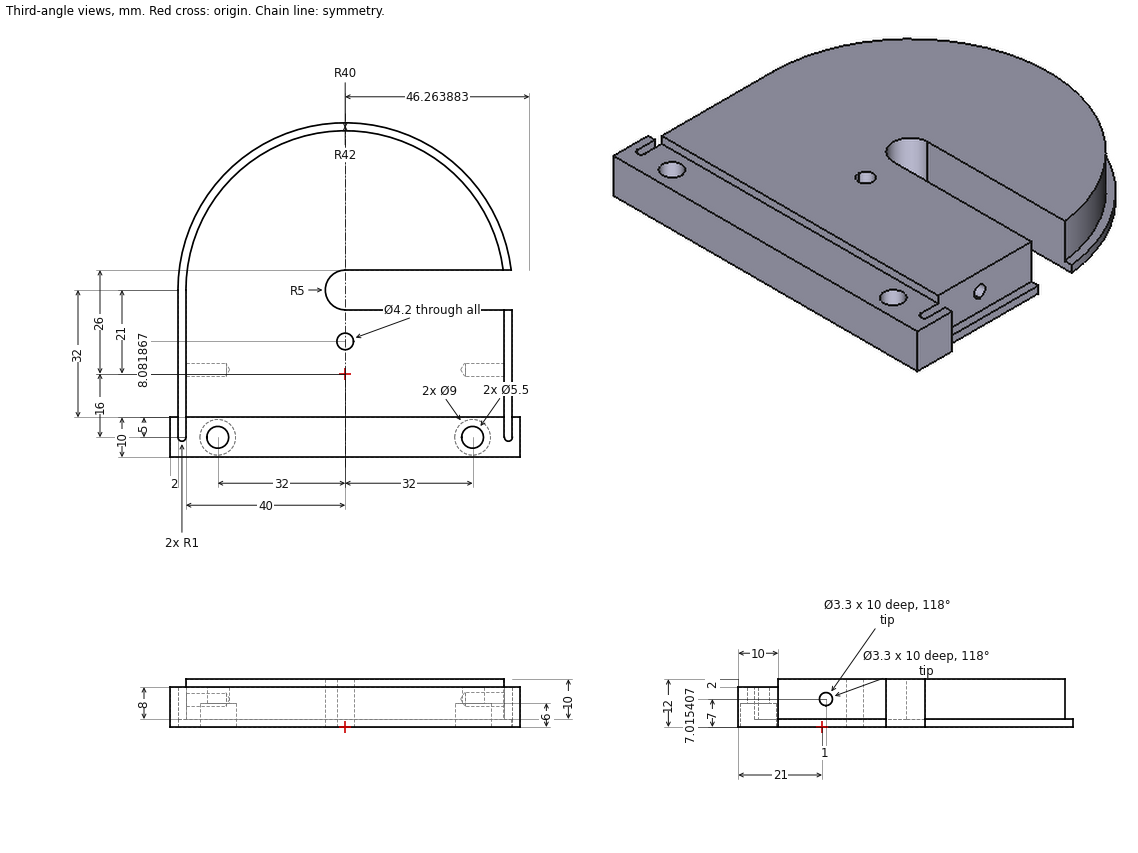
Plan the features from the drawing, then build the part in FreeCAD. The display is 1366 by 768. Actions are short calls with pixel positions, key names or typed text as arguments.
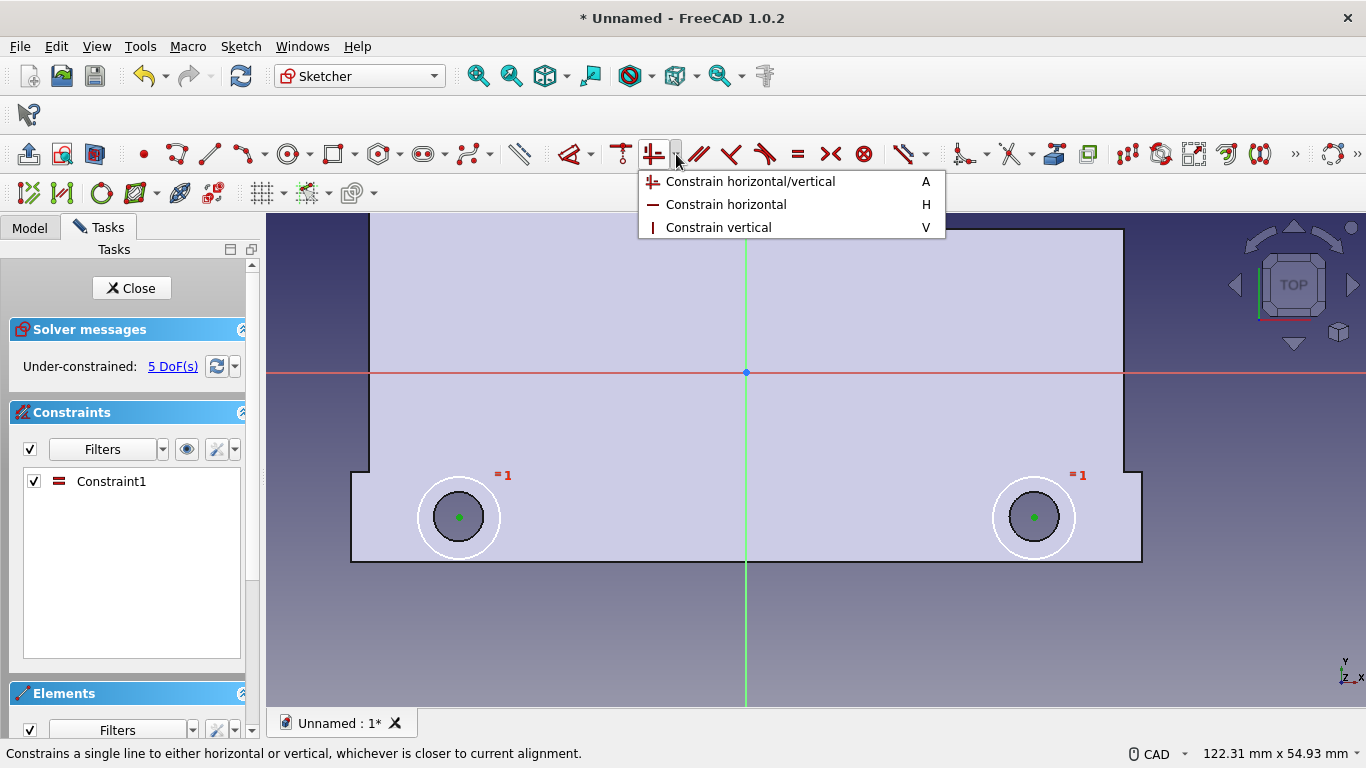
click(792, 204)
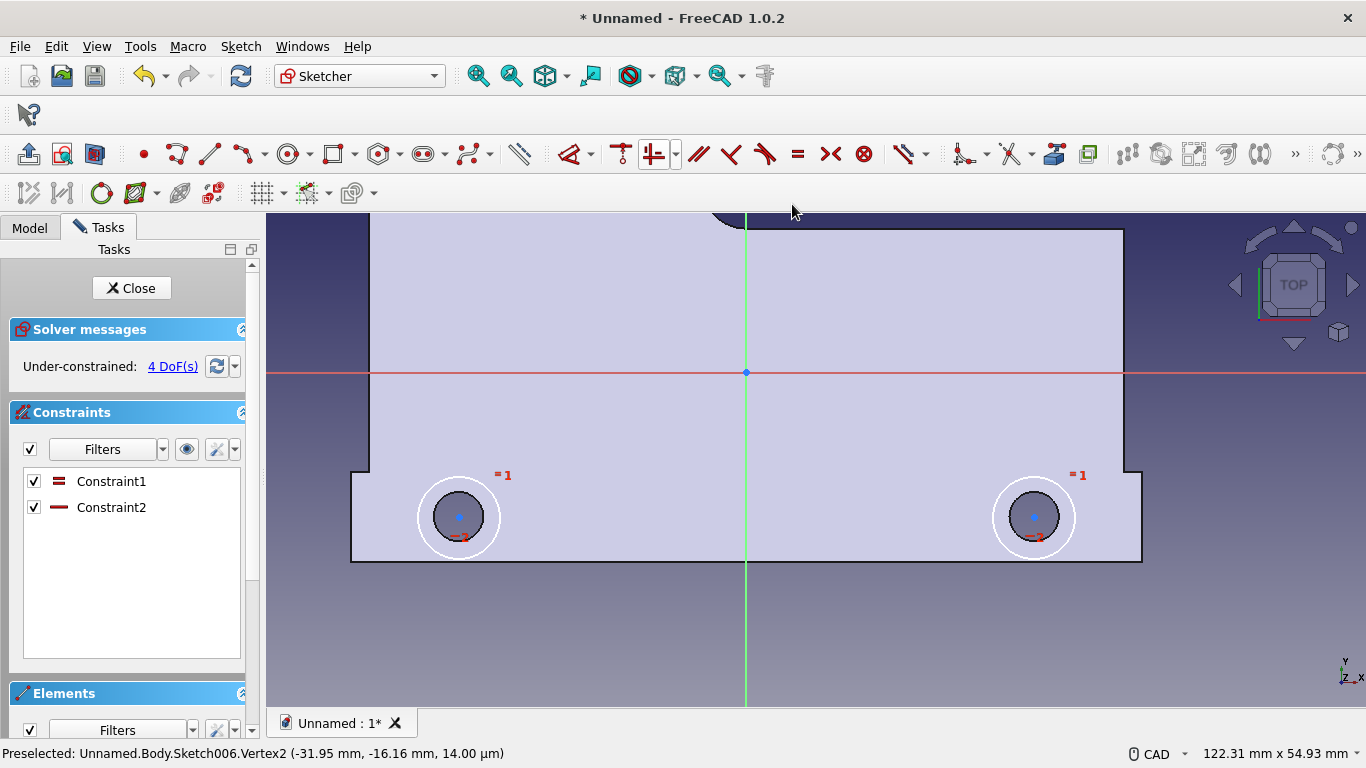
key(d)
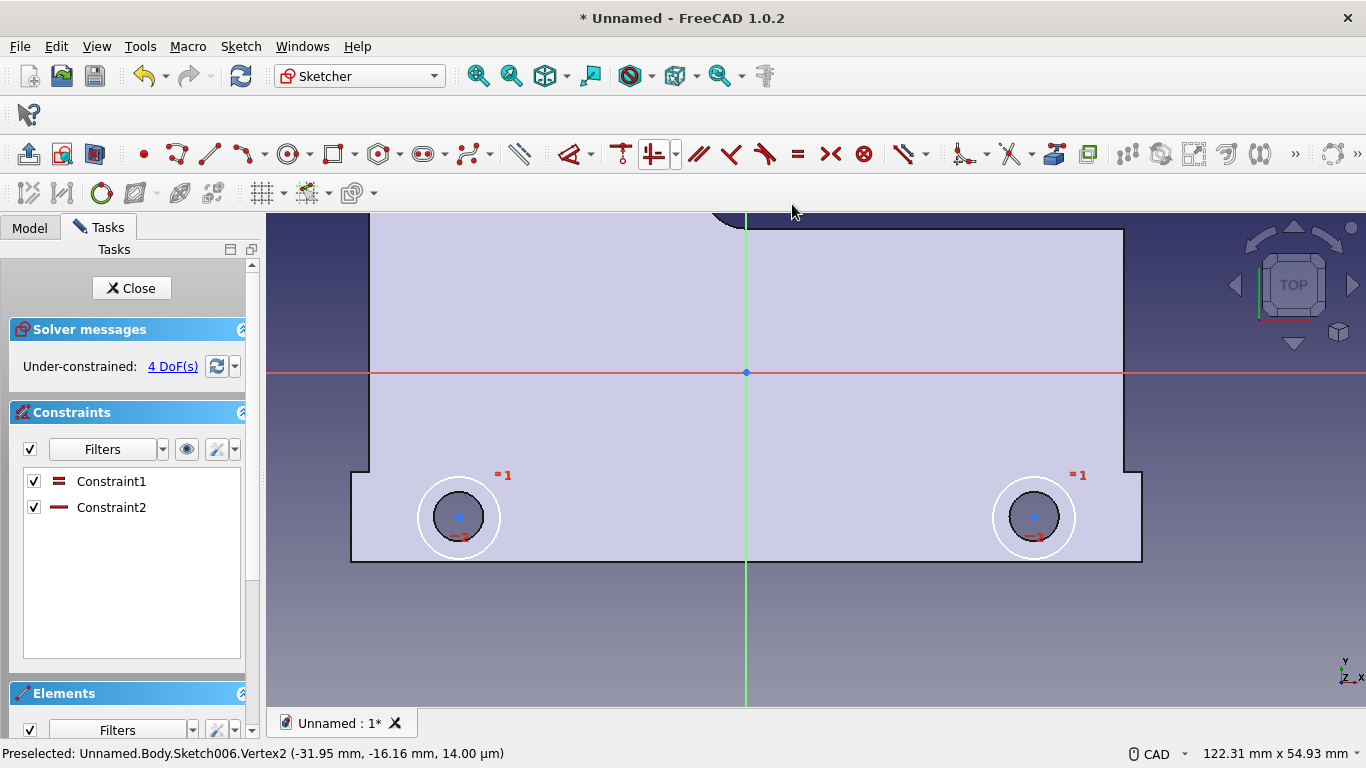
click(1063, 489)
click(1086, 466)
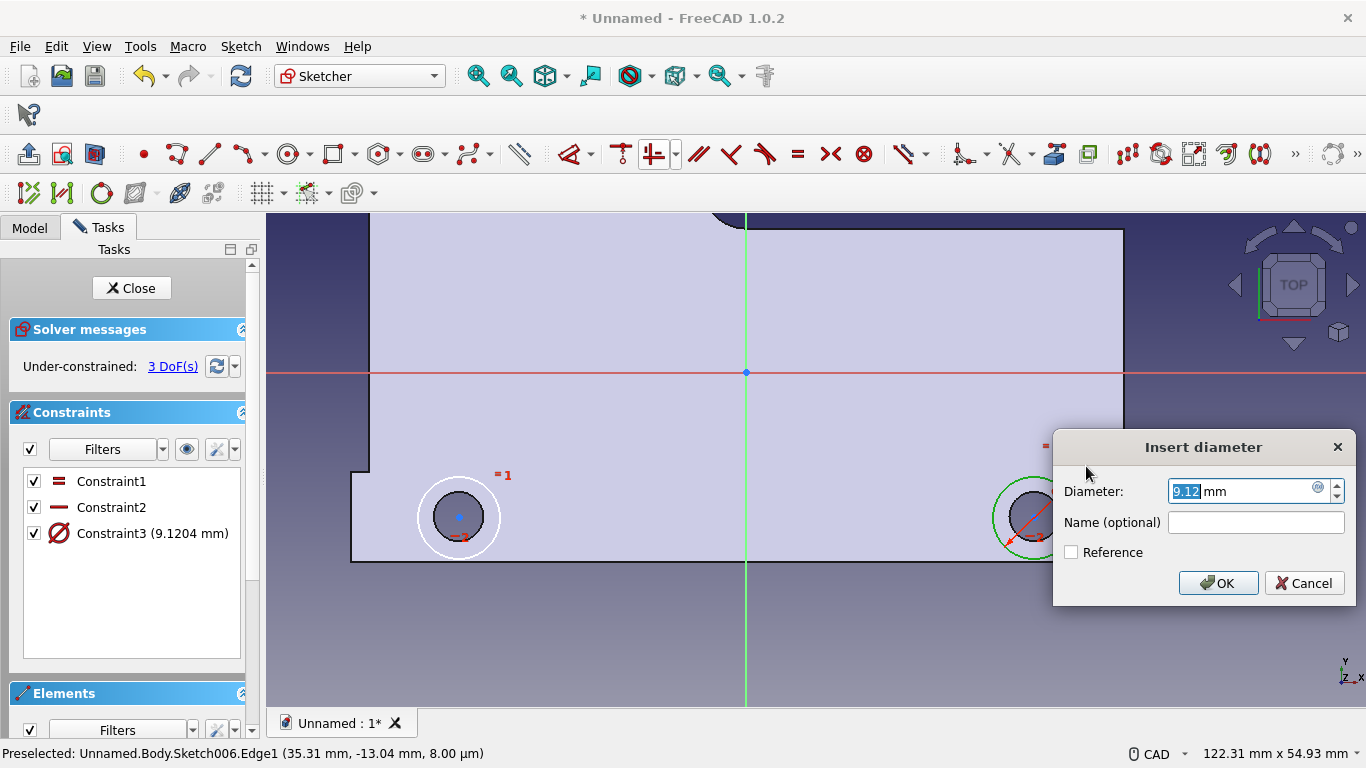
text(9)
key(Return)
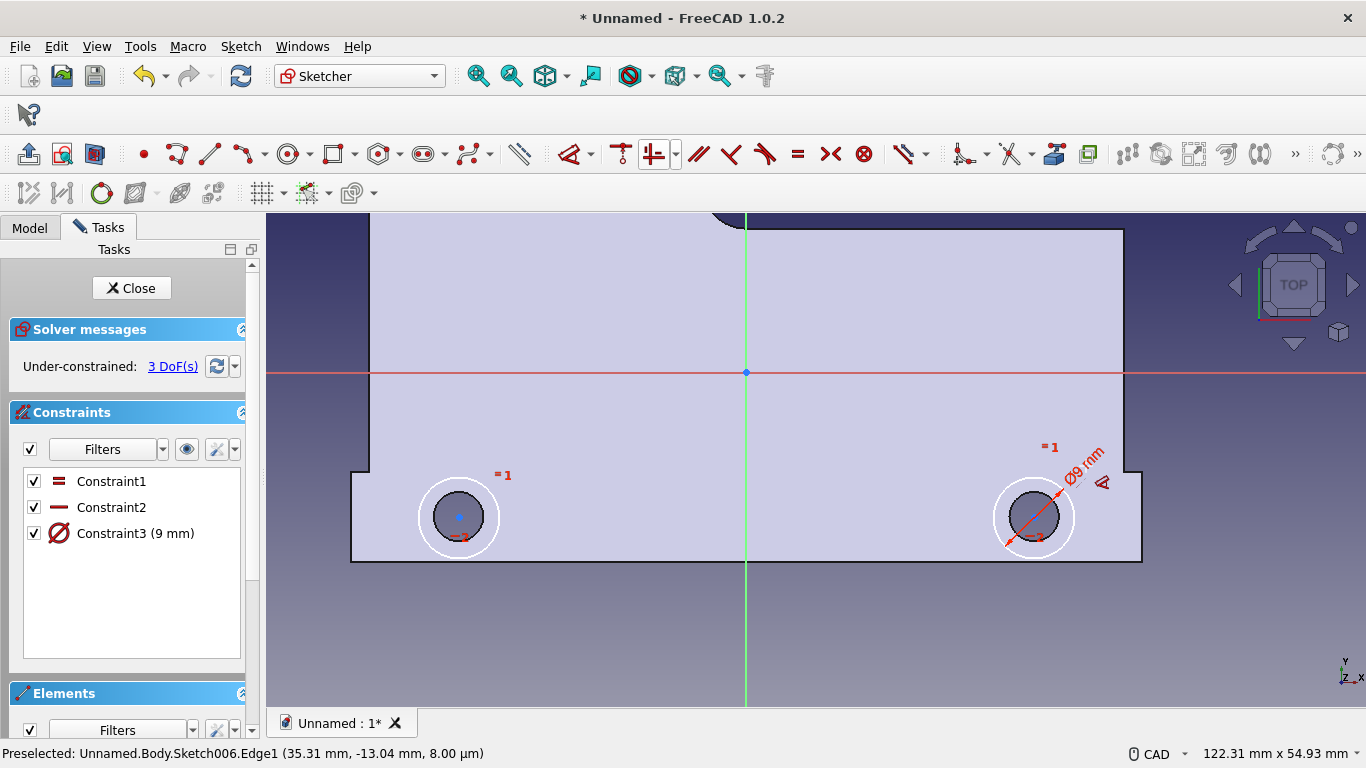
click(1034, 518)
click(890, 339)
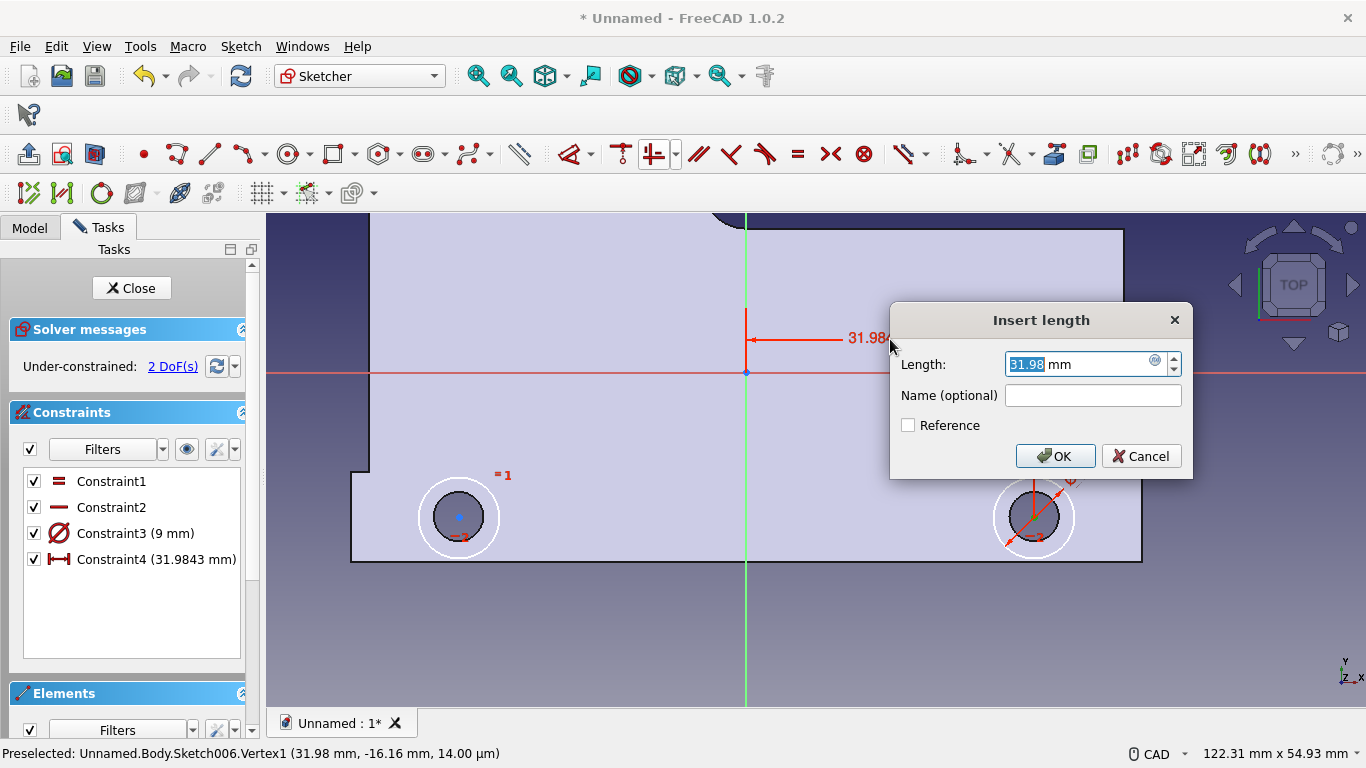
text(32)
key(Return)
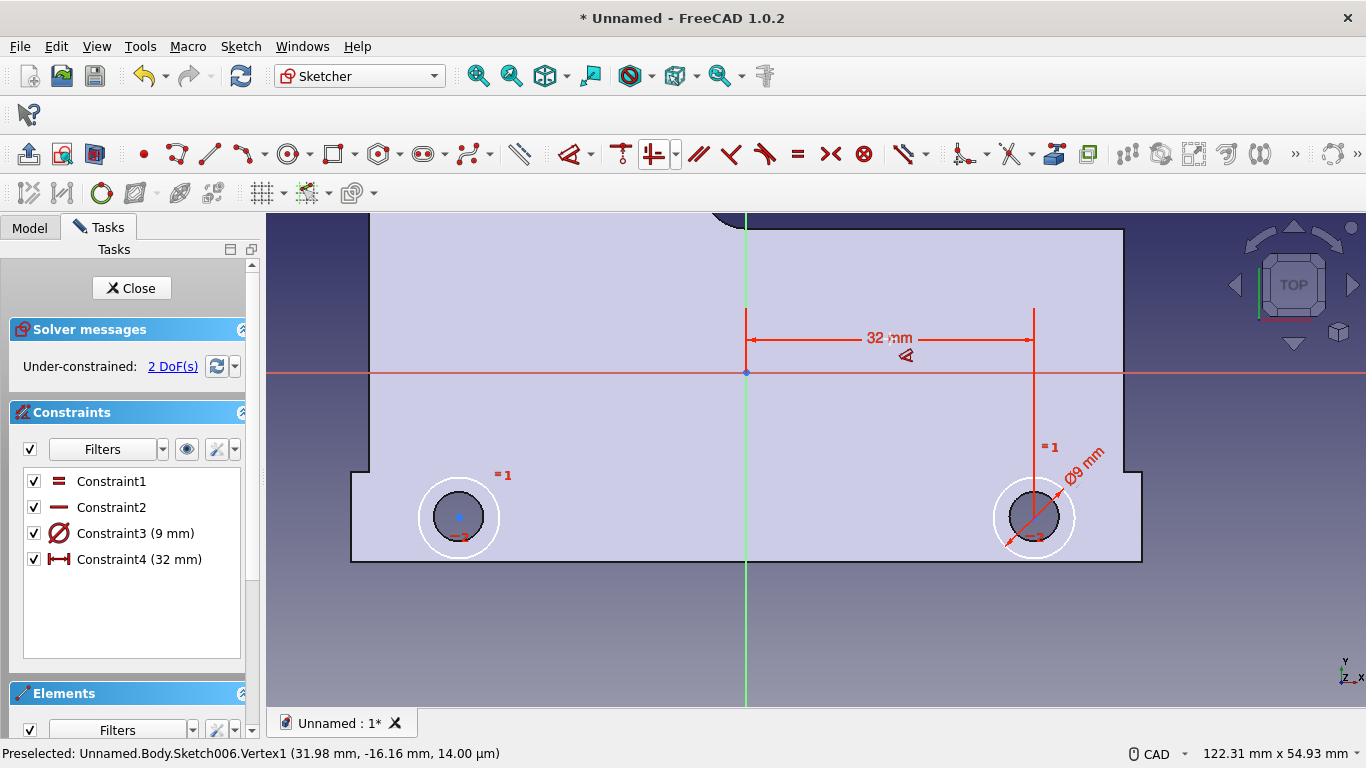
click(1034, 518)
click(1068, 445)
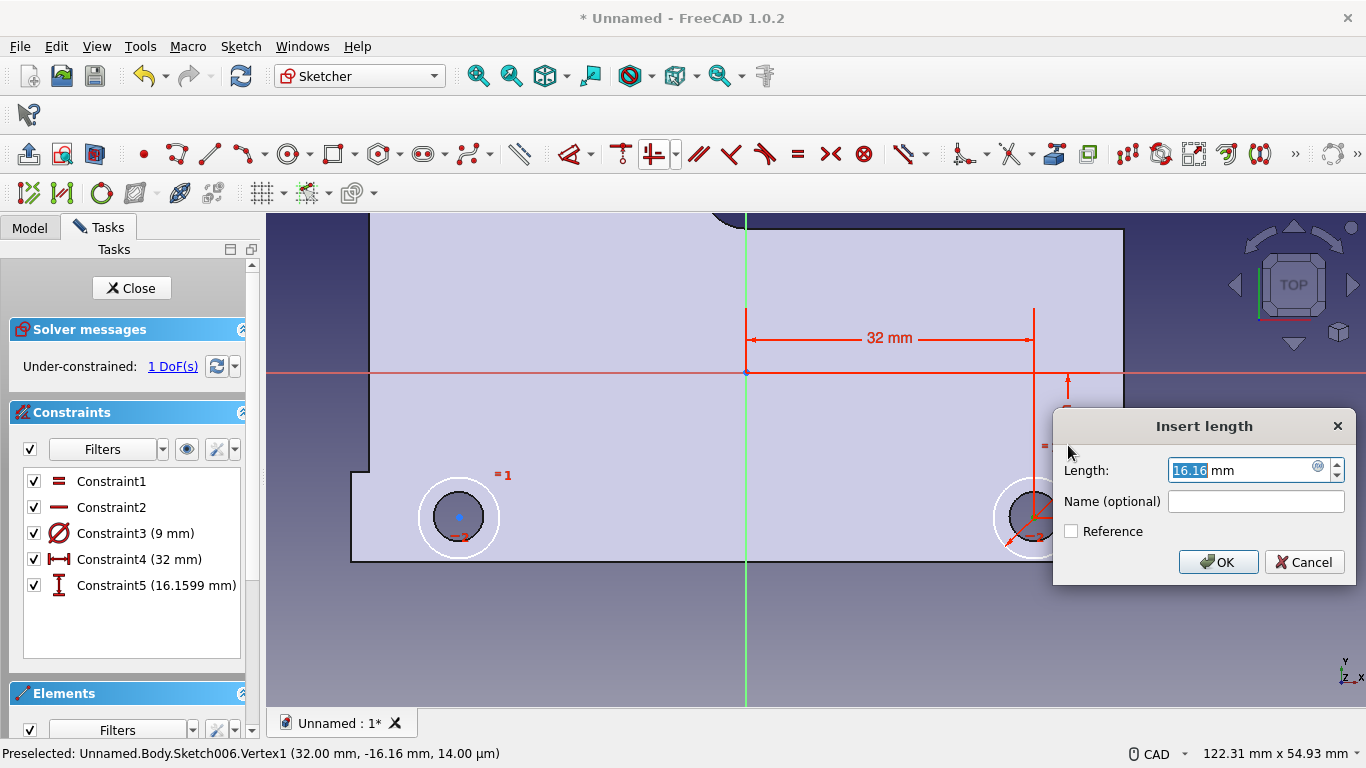
text(16)
key(Return)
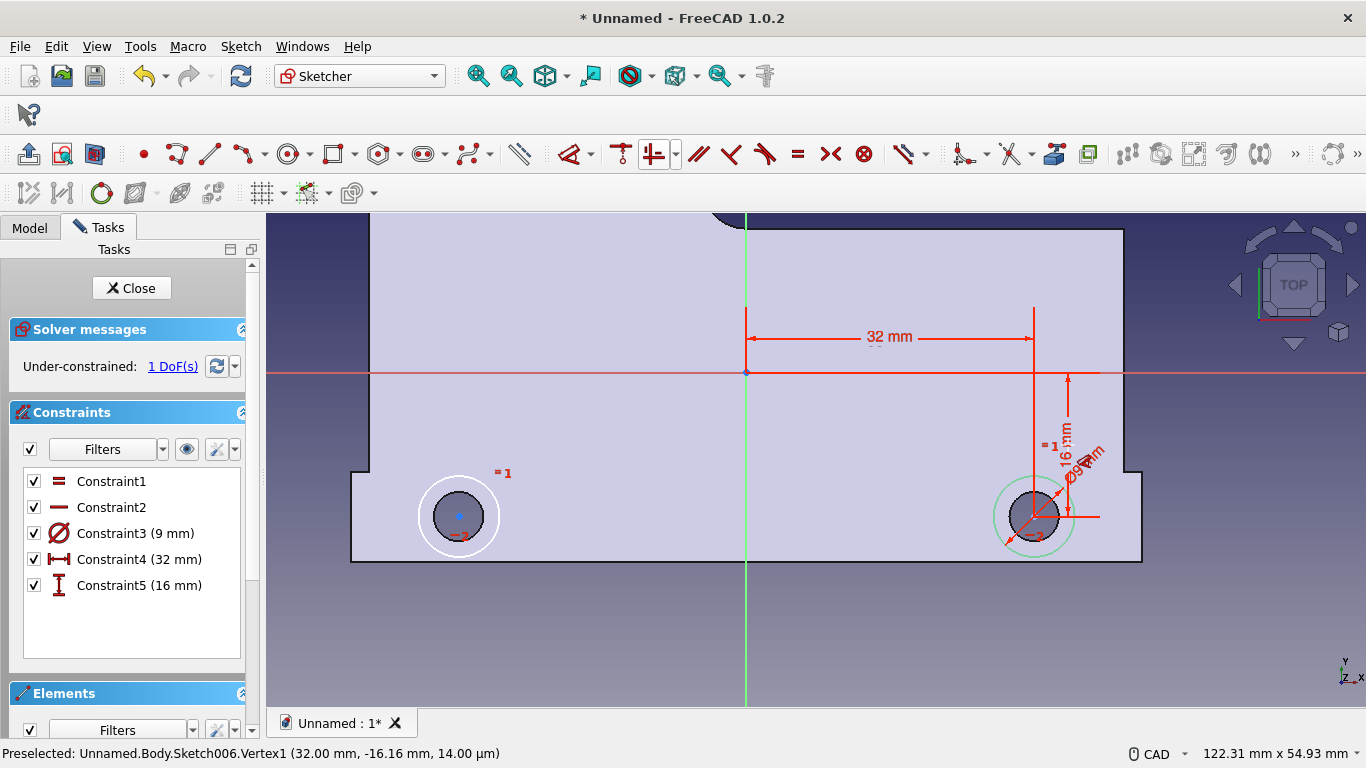
click(459, 517)
click(603, 339)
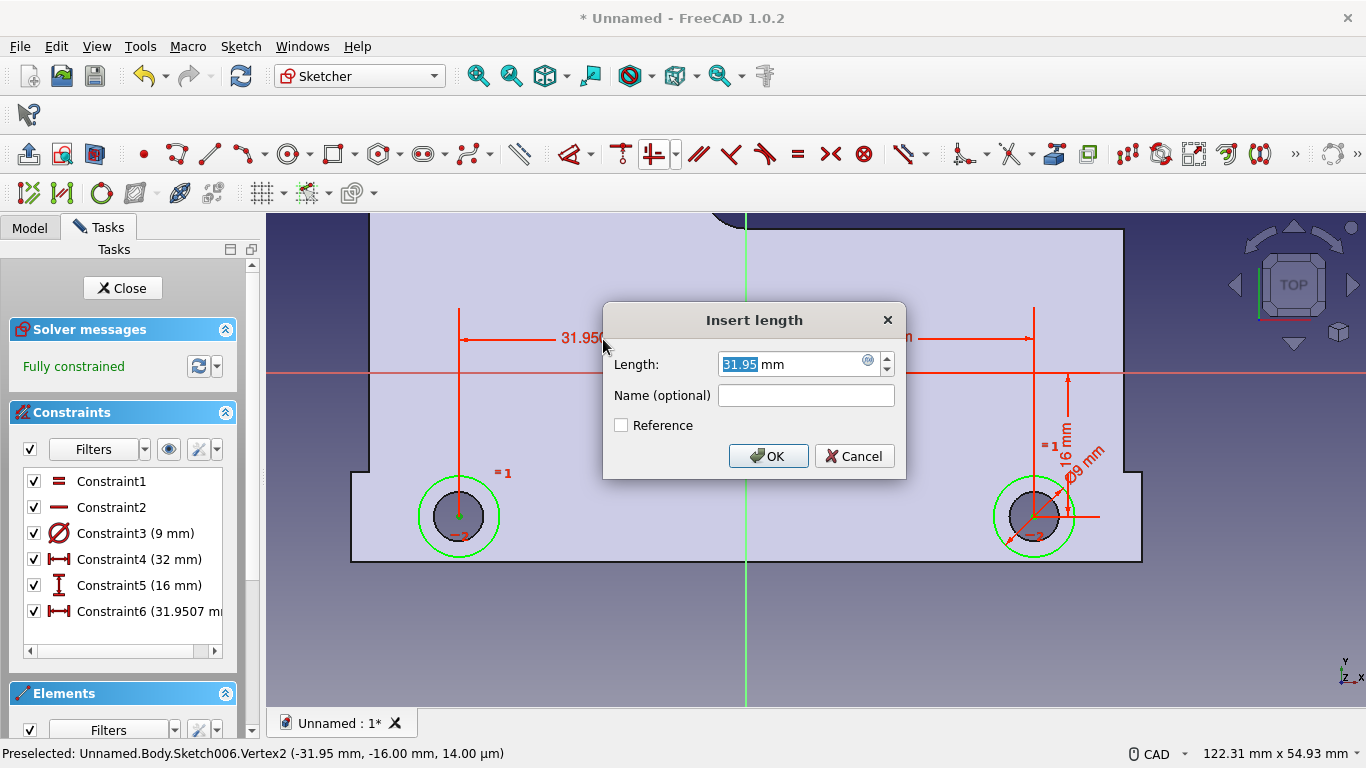
text(32)
key(Return)
key(Escape)